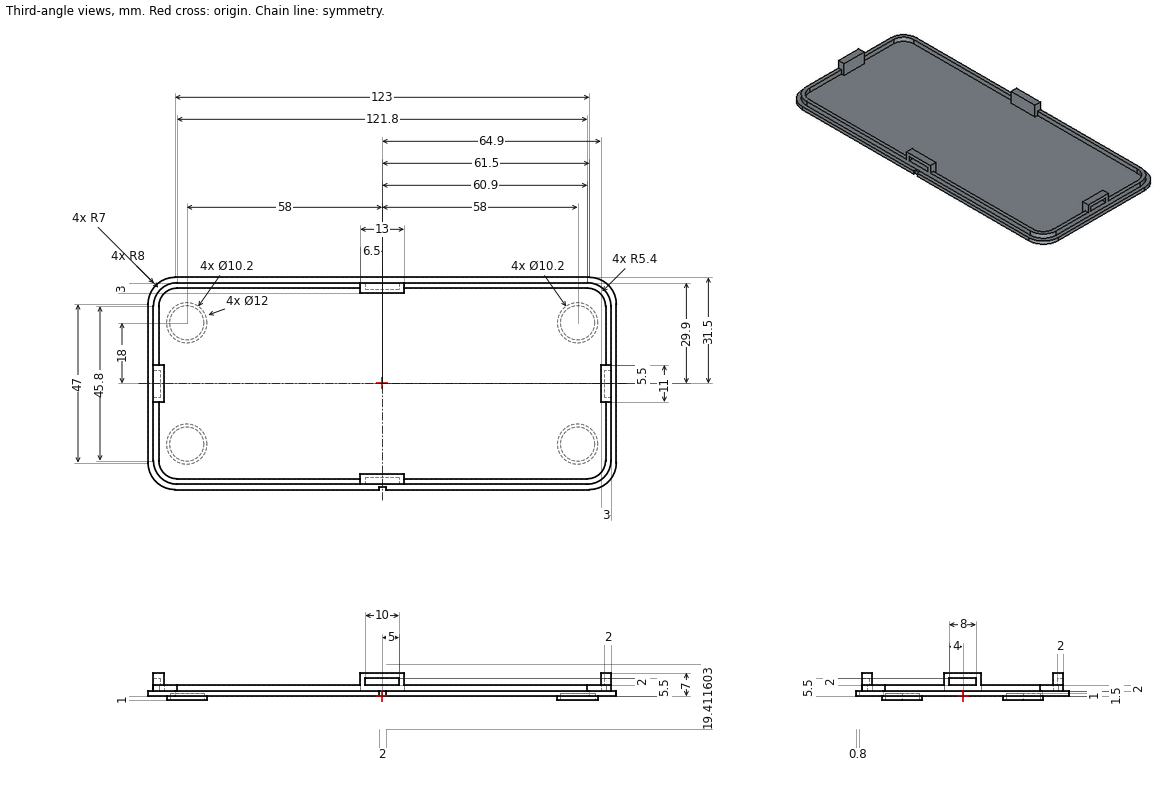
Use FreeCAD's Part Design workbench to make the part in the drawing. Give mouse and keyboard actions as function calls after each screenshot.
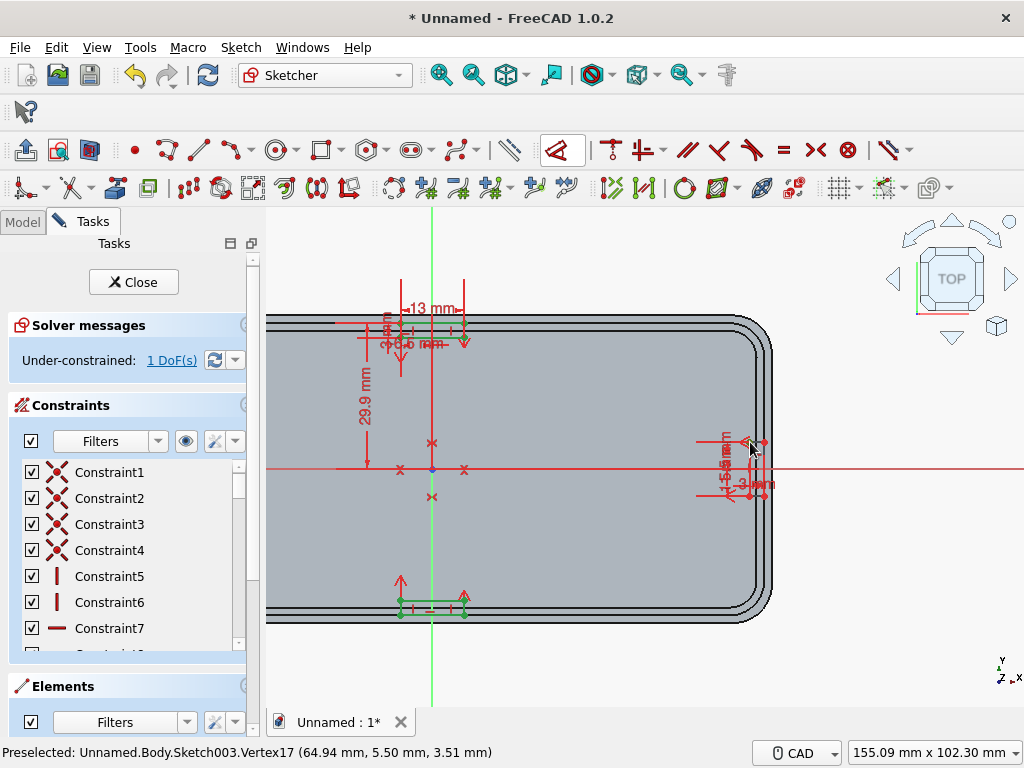
key(l)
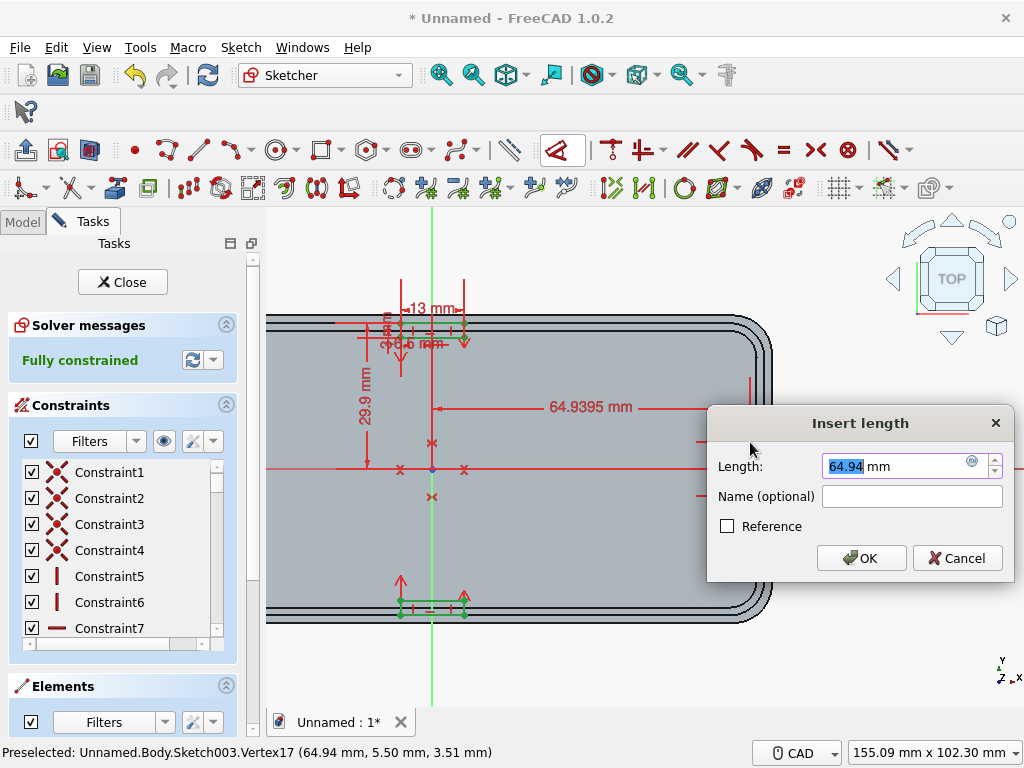
text(64.9)
key(Return)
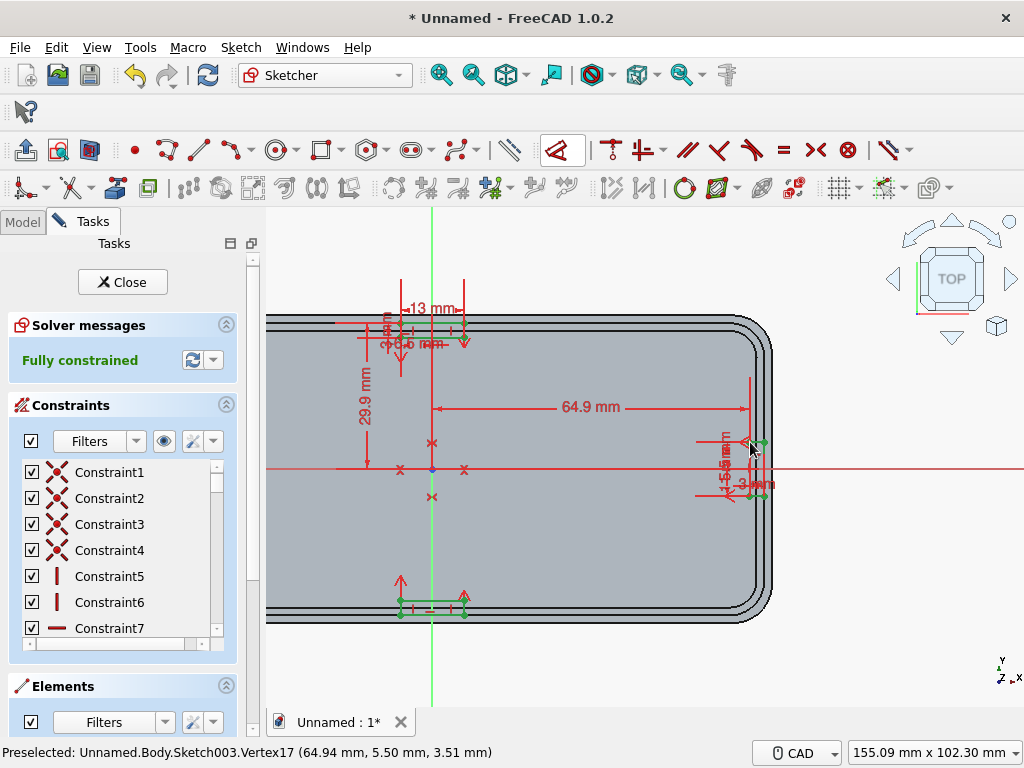
click(123, 282)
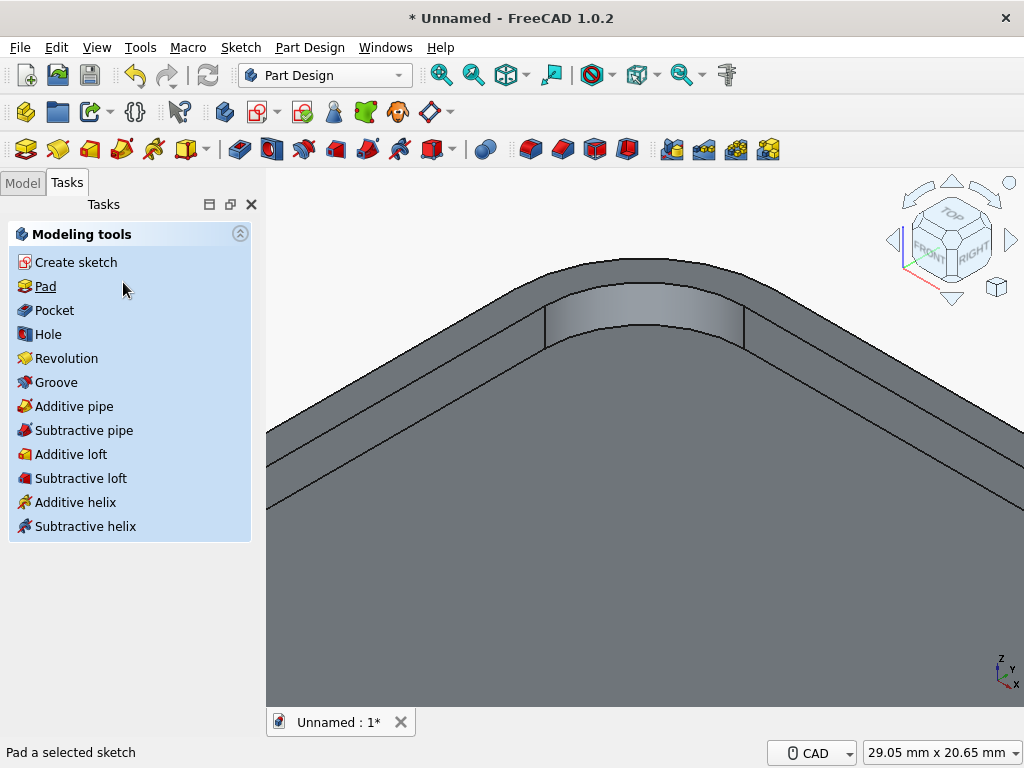
click(26, 150)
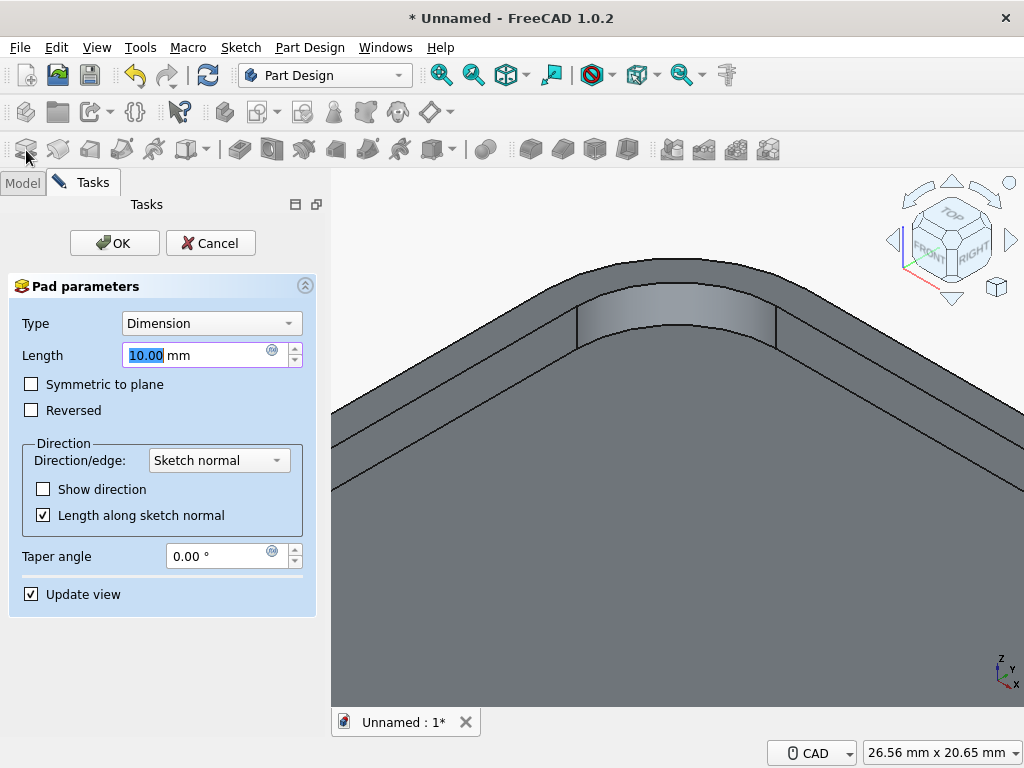
text(7)
key(Tab)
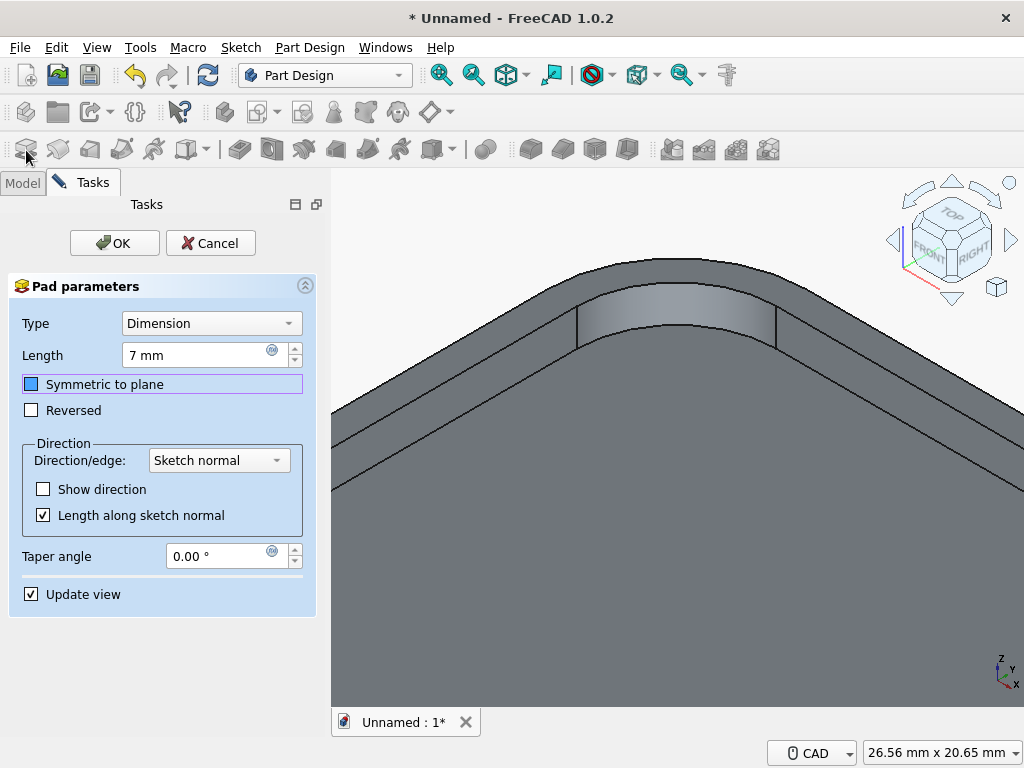
click(30, 384)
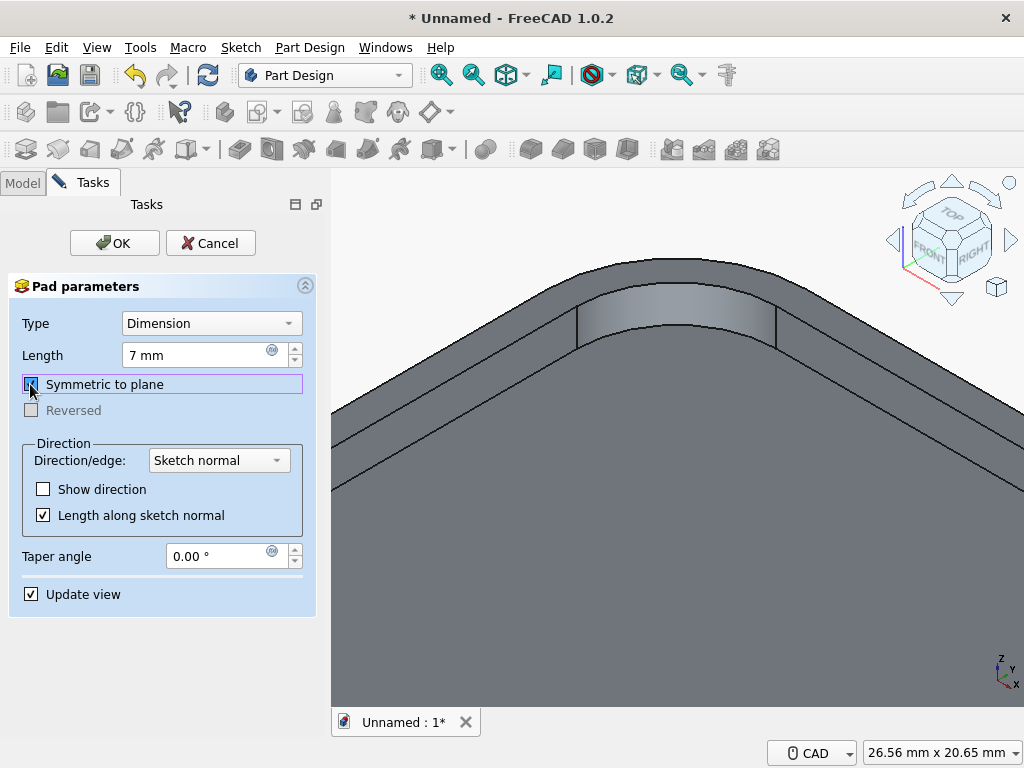
click(115, 243)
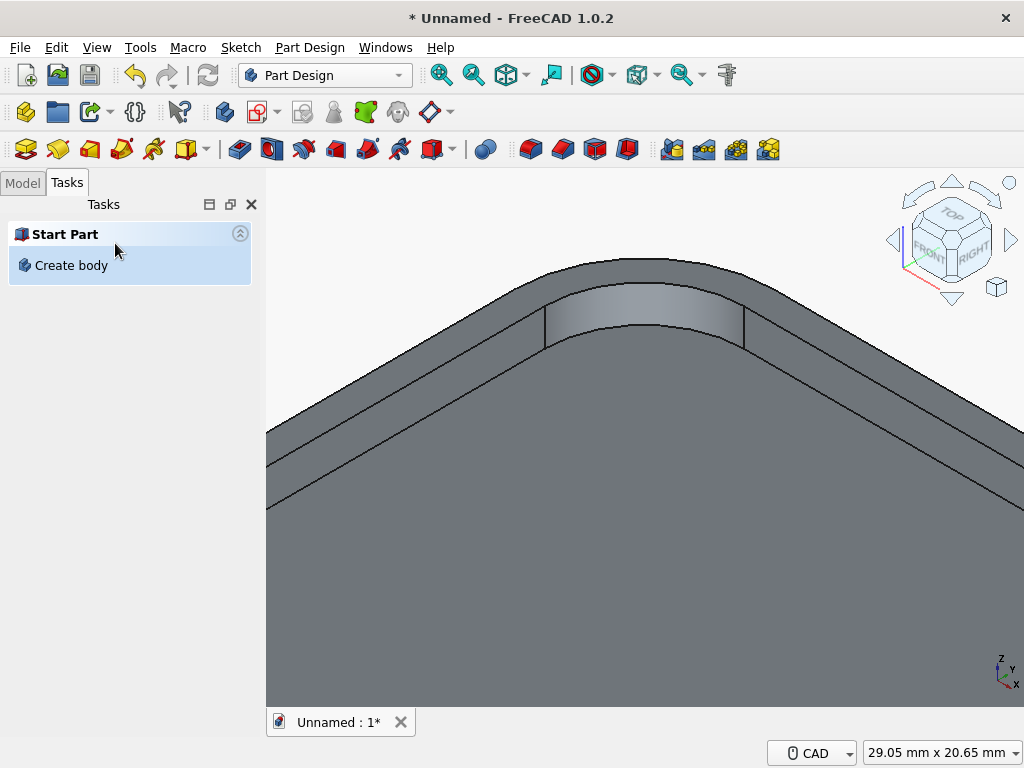
click(442, 76)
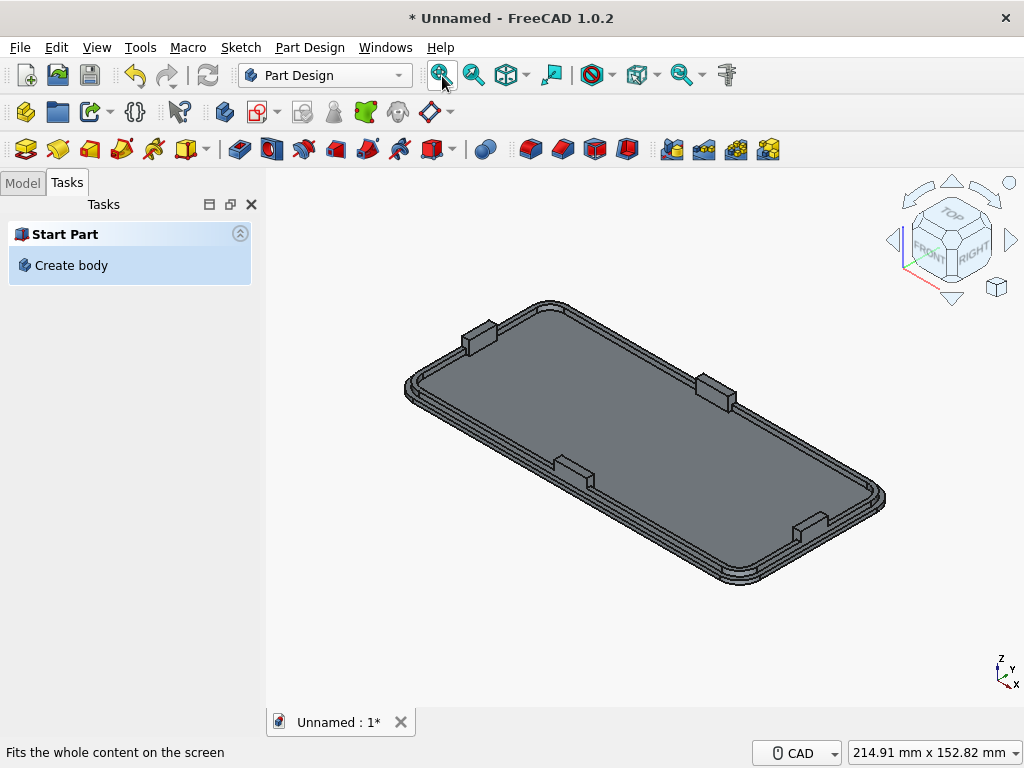
key(4)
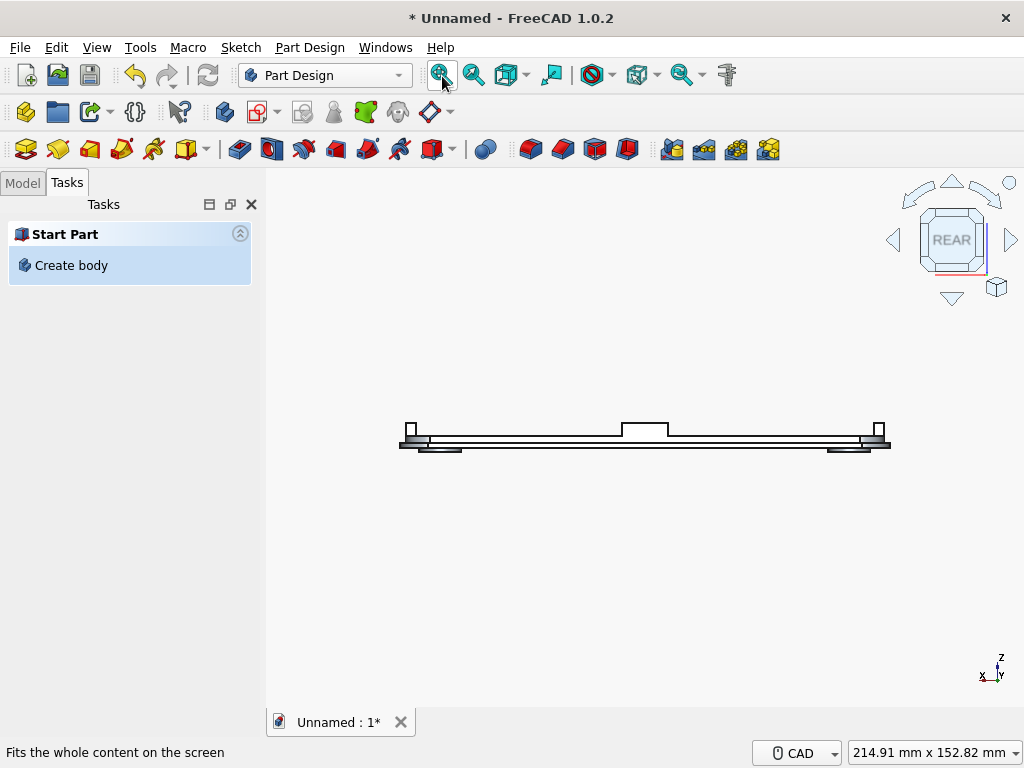
click(645, 432)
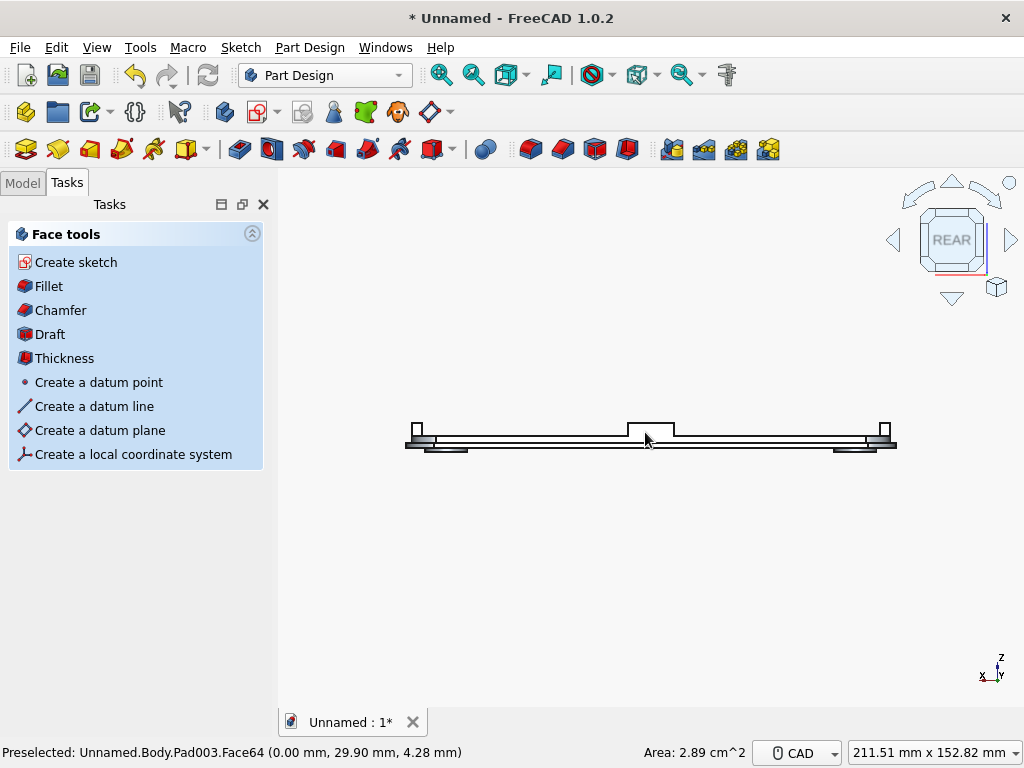
click(258, 112)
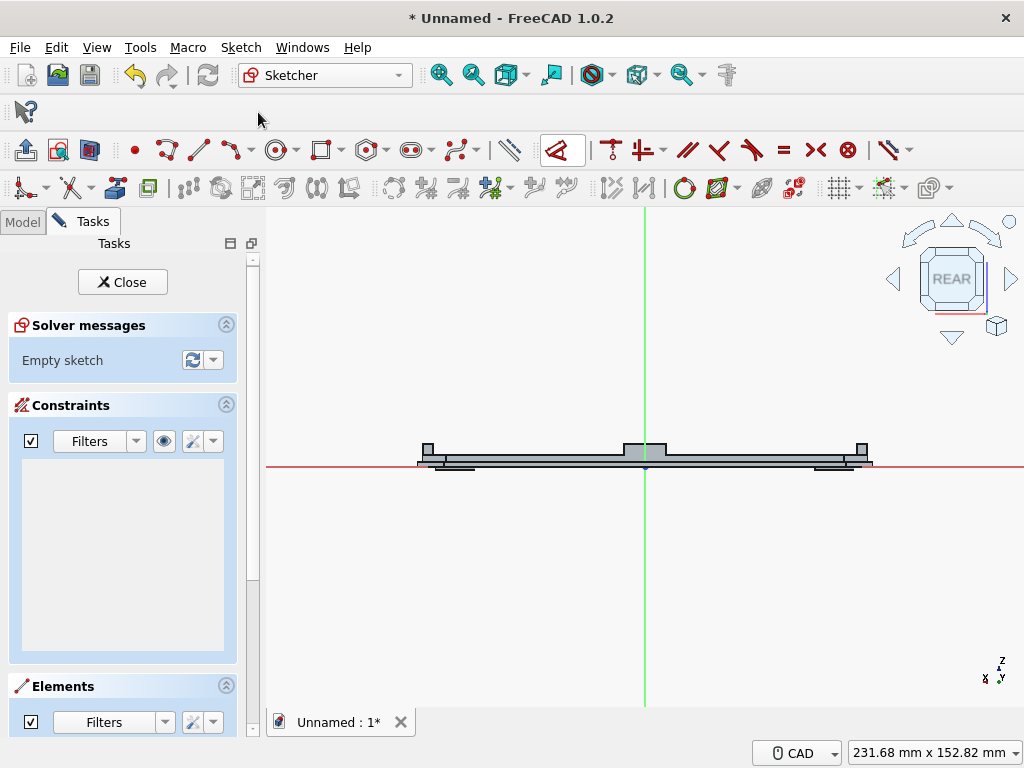
key(q)
key(s)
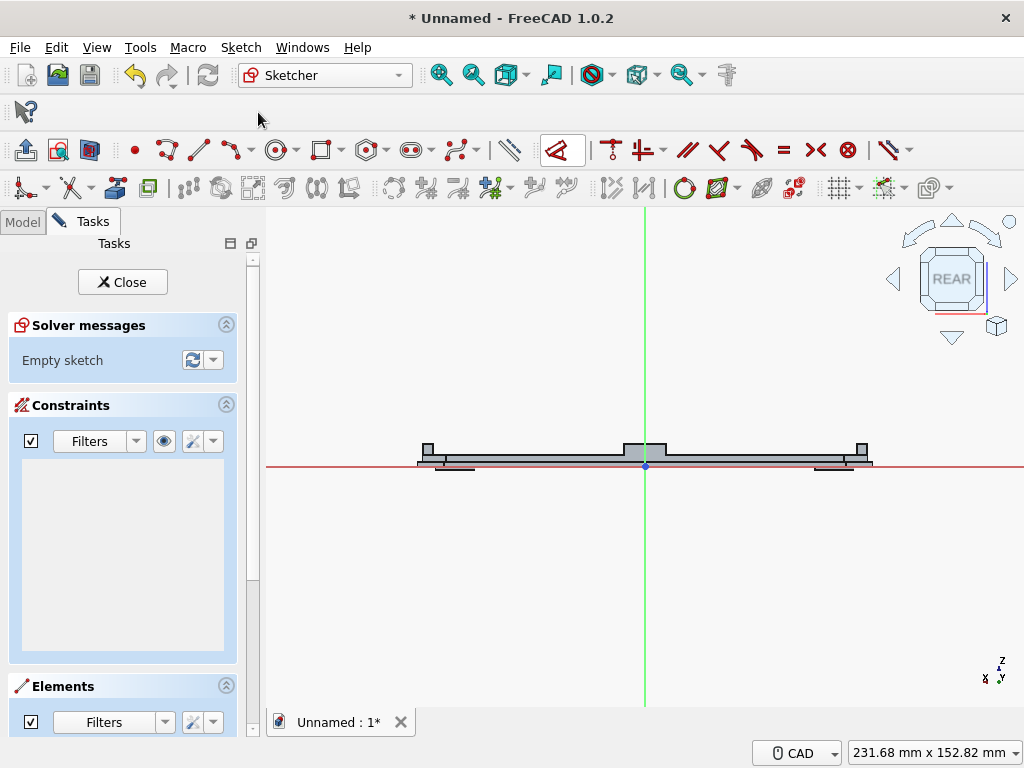
scroll(650, 458, up, 13)